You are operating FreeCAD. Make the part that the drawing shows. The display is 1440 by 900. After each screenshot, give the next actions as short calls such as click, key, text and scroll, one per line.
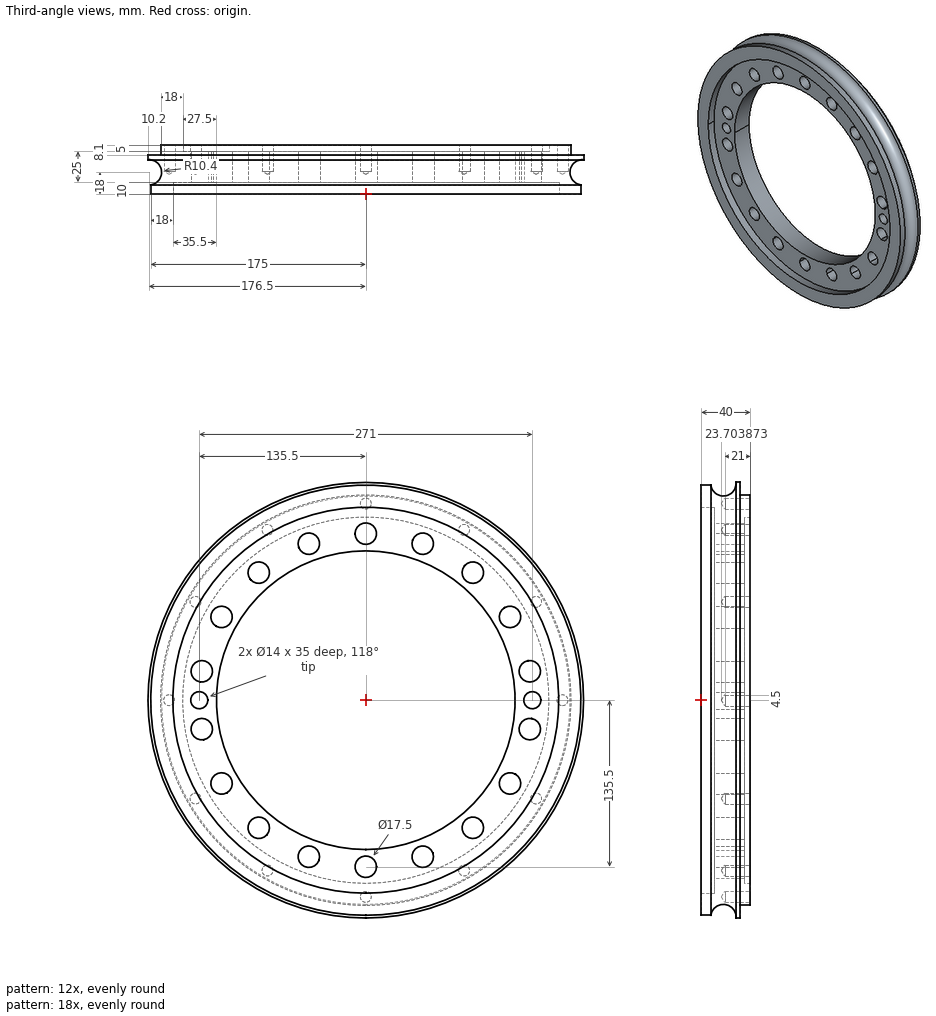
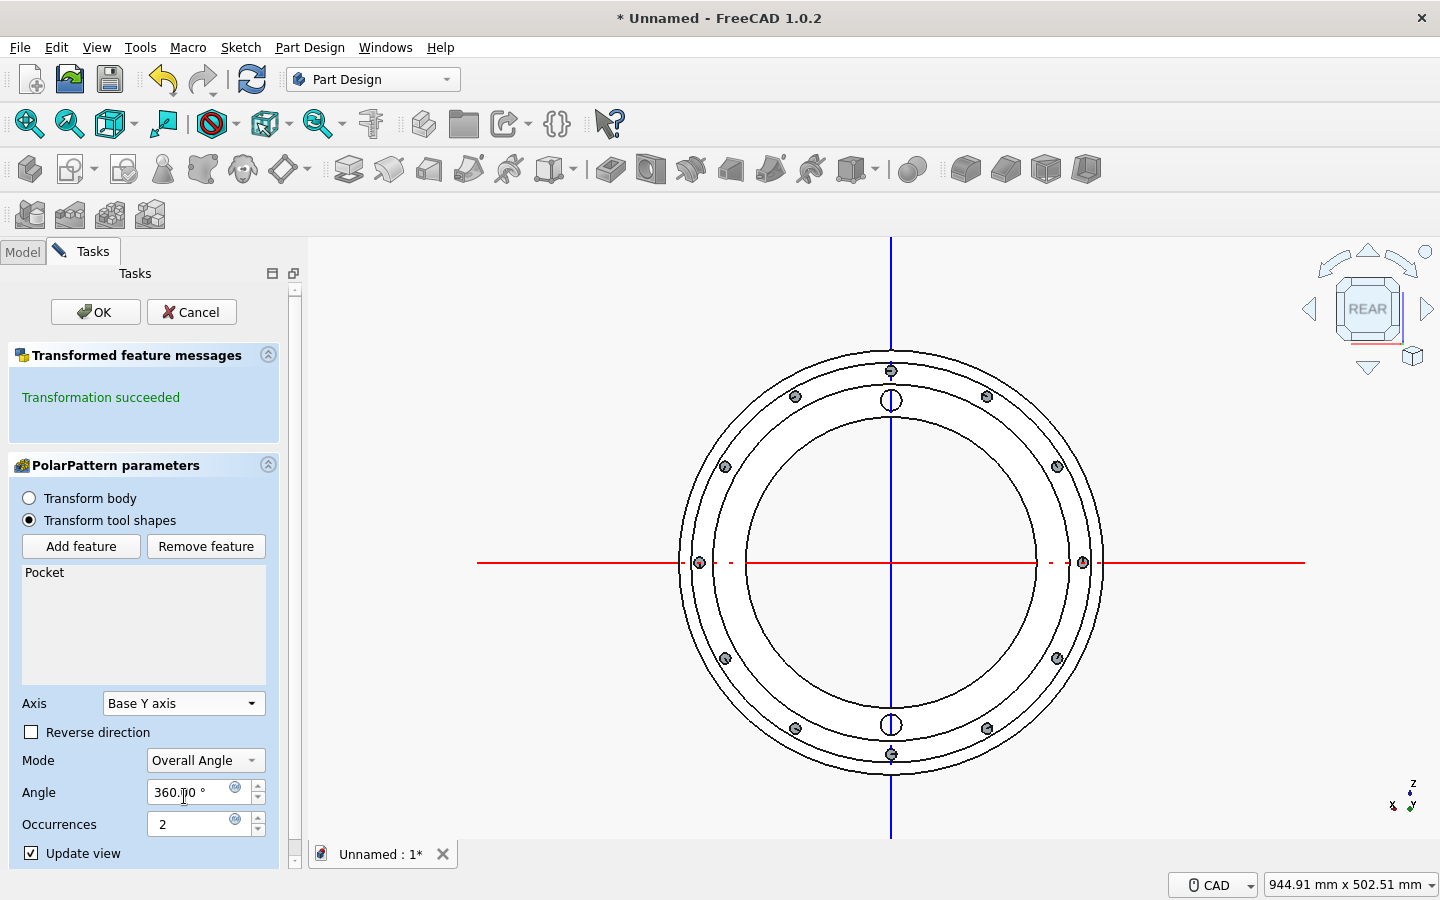
triple_click(198, 824)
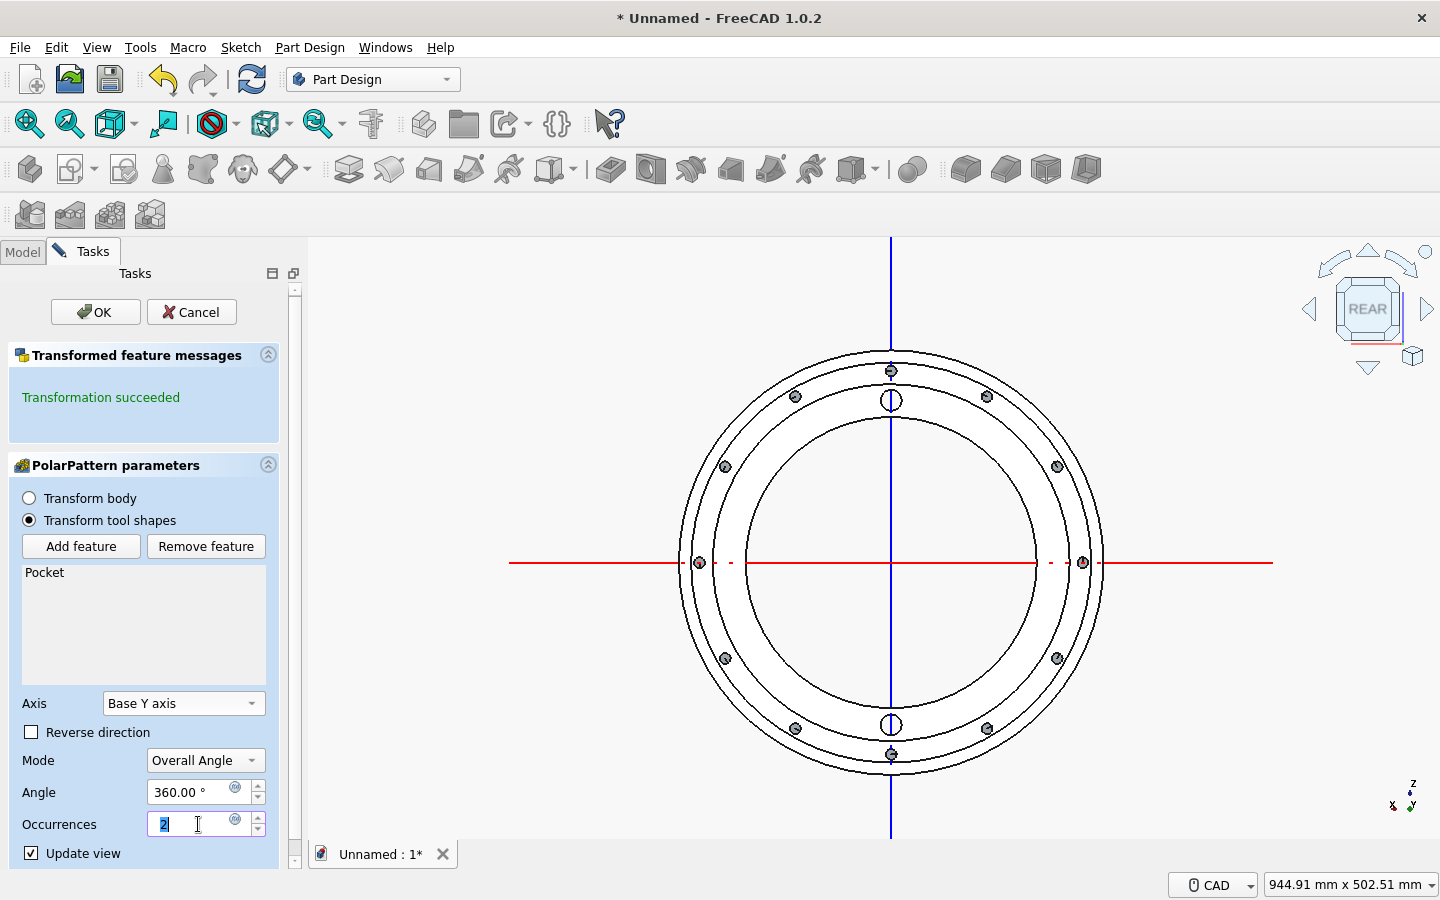
text(18)
key(Tab)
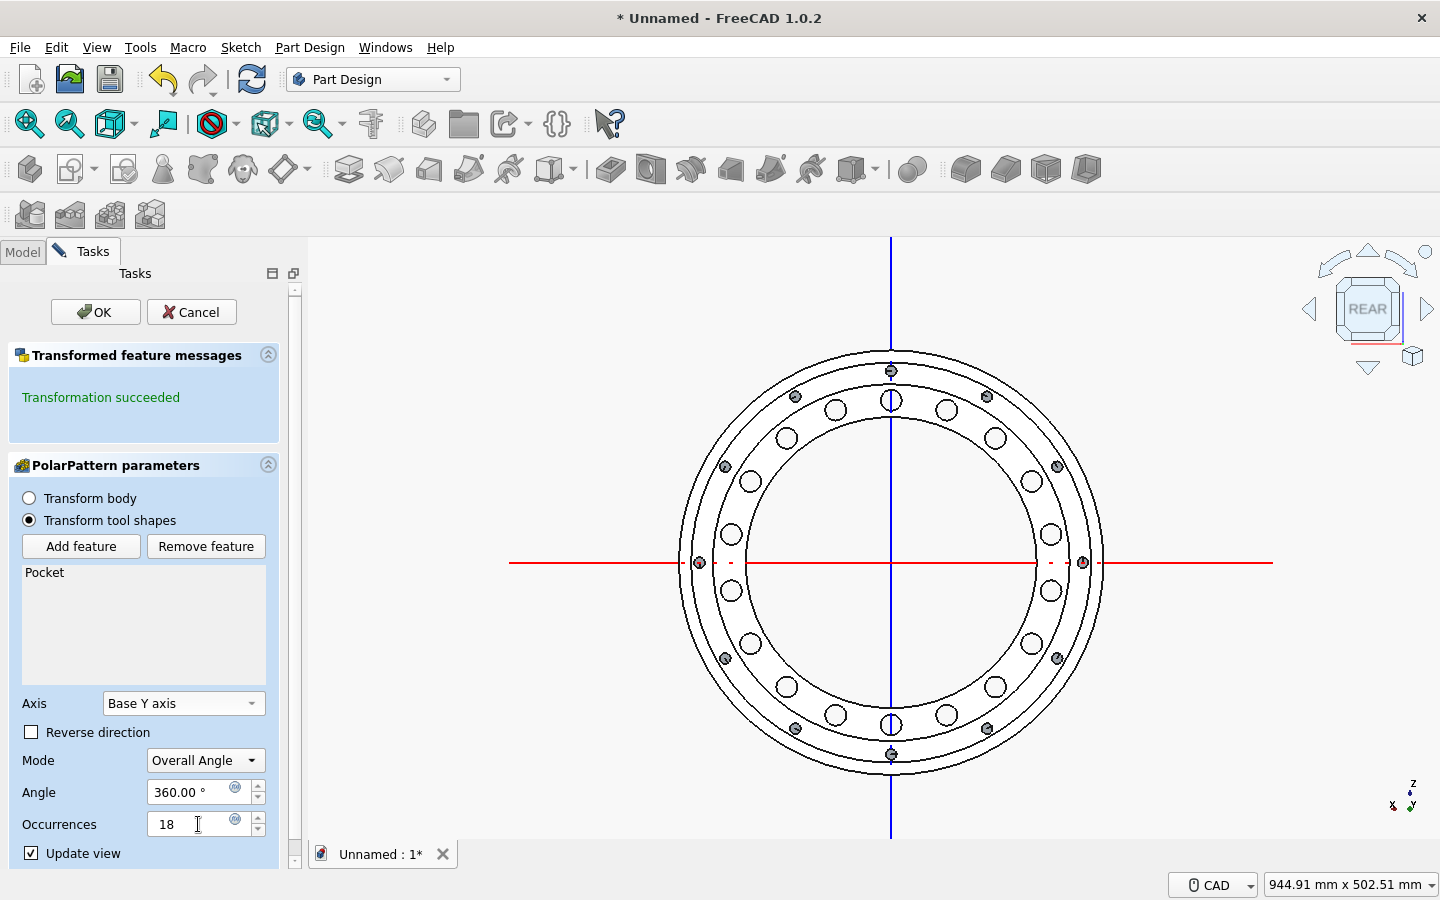
click(96, 312)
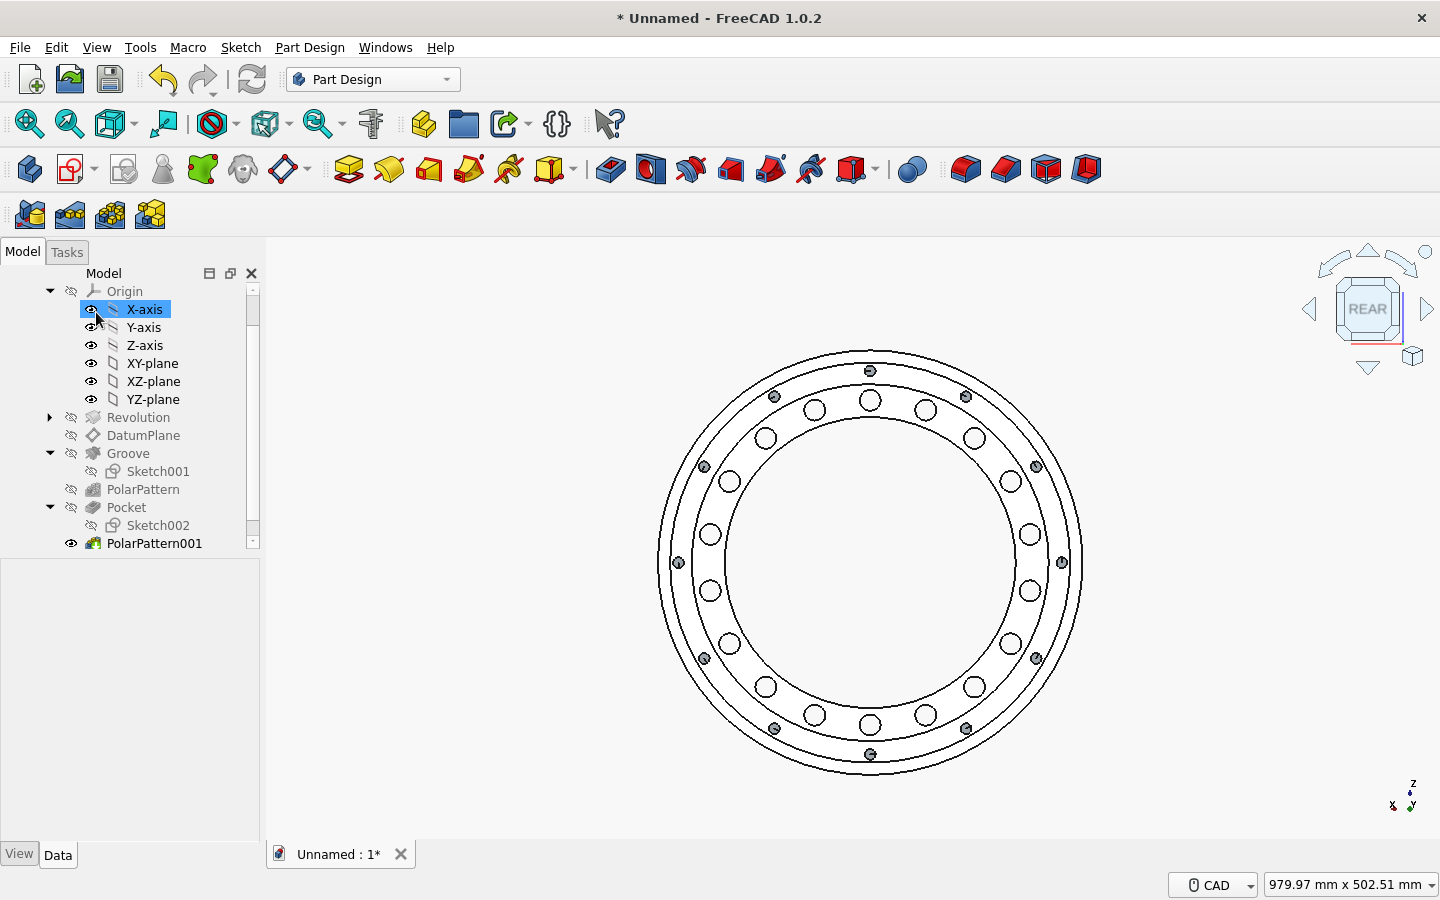
click(717, 613)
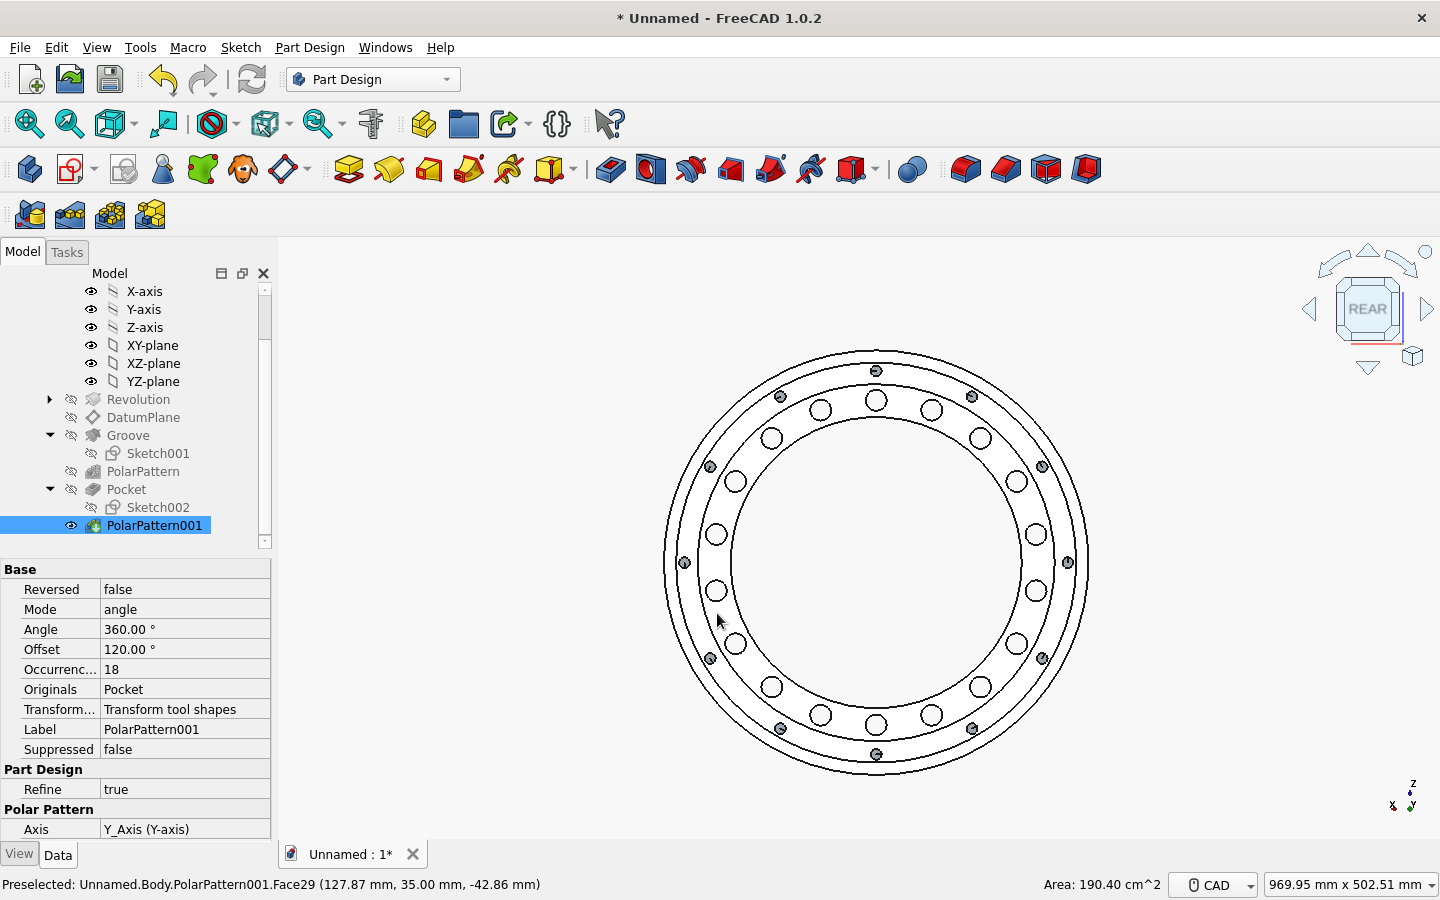
click(70, 170)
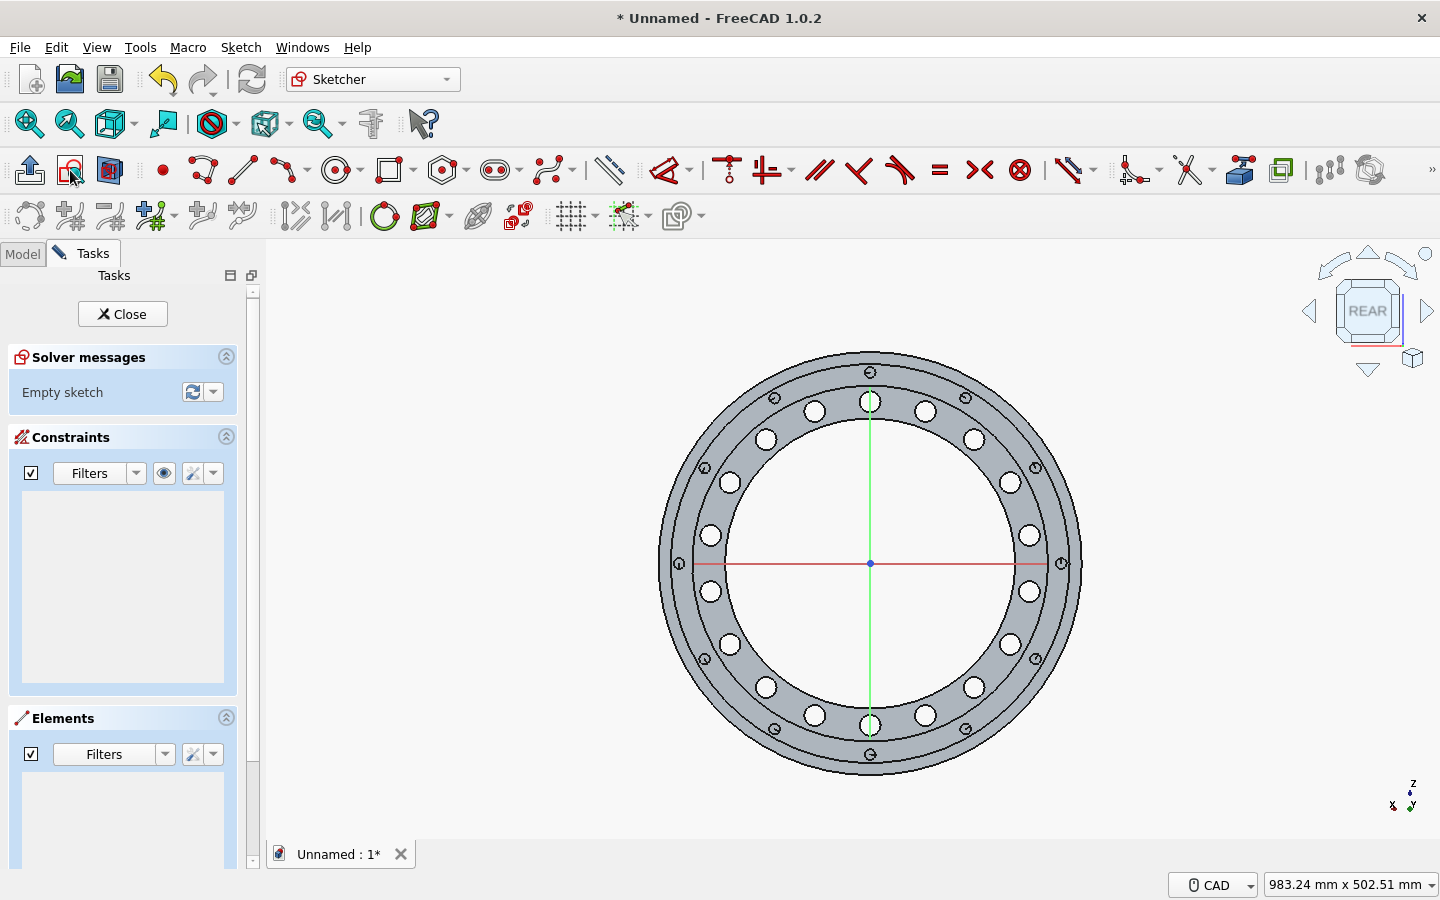
scroll(940, 584, up, 4)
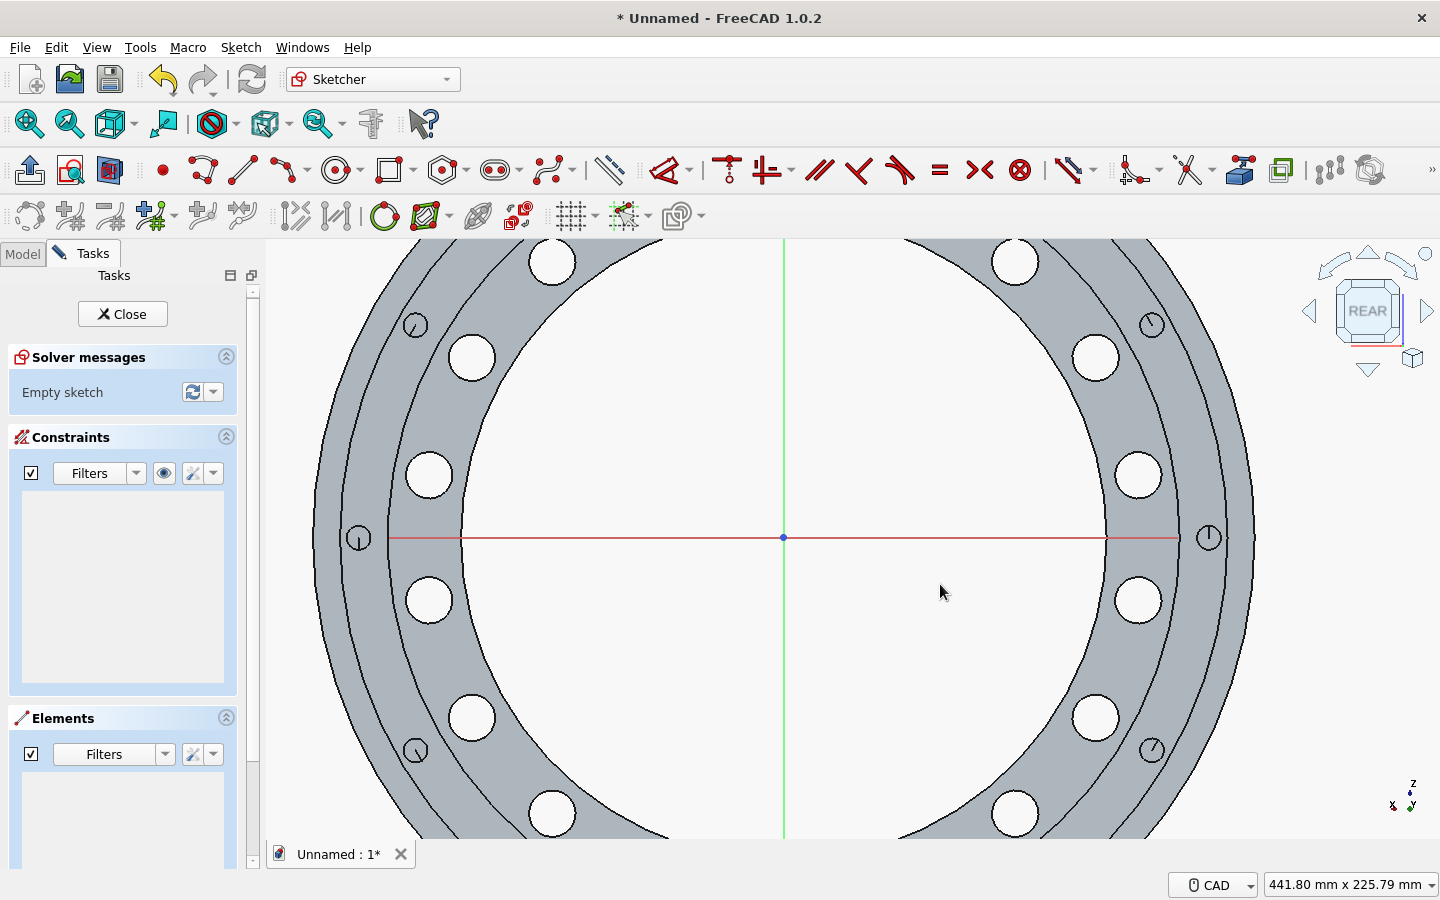
click(336, 170)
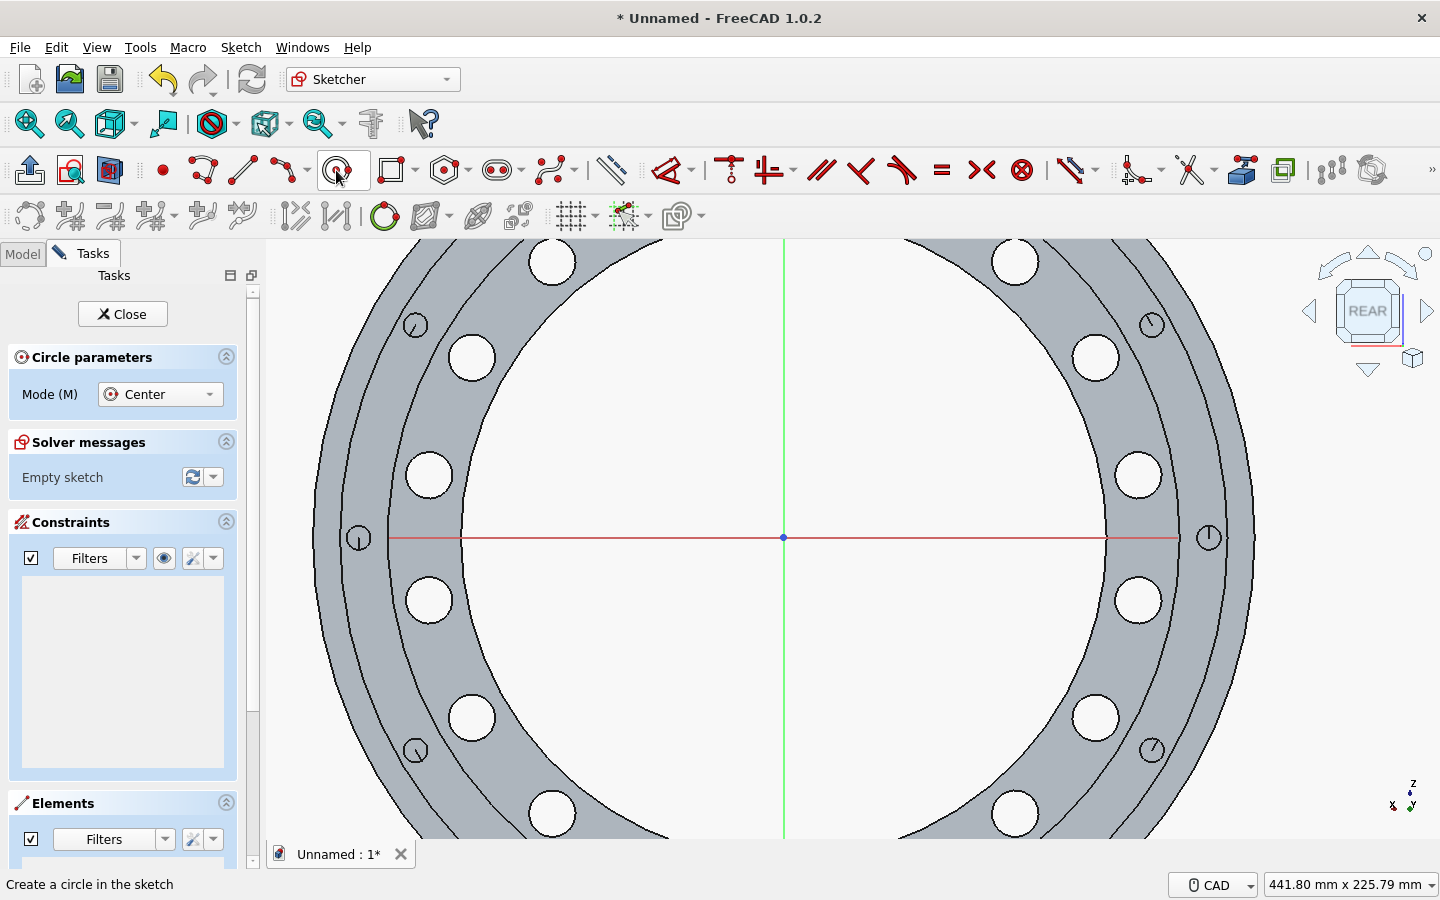
click(1144, 538)
move(1150, 520)